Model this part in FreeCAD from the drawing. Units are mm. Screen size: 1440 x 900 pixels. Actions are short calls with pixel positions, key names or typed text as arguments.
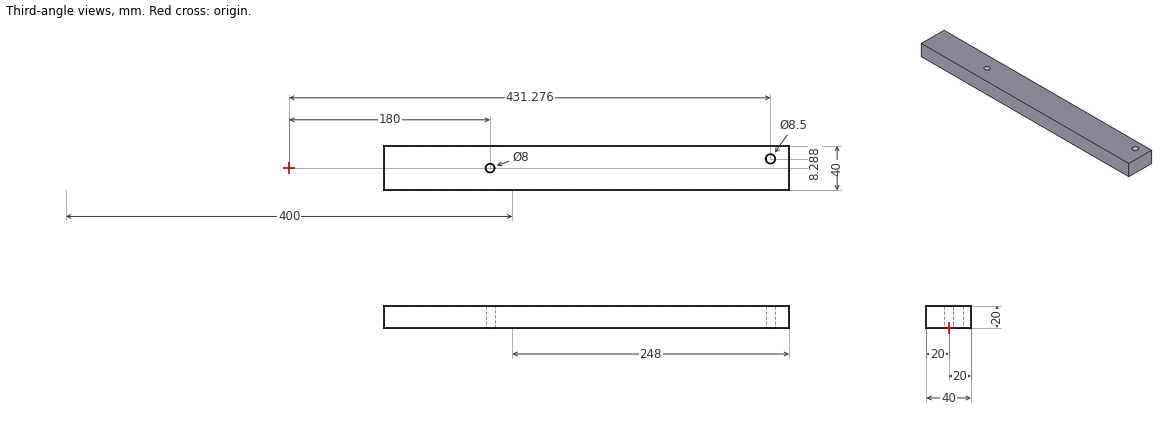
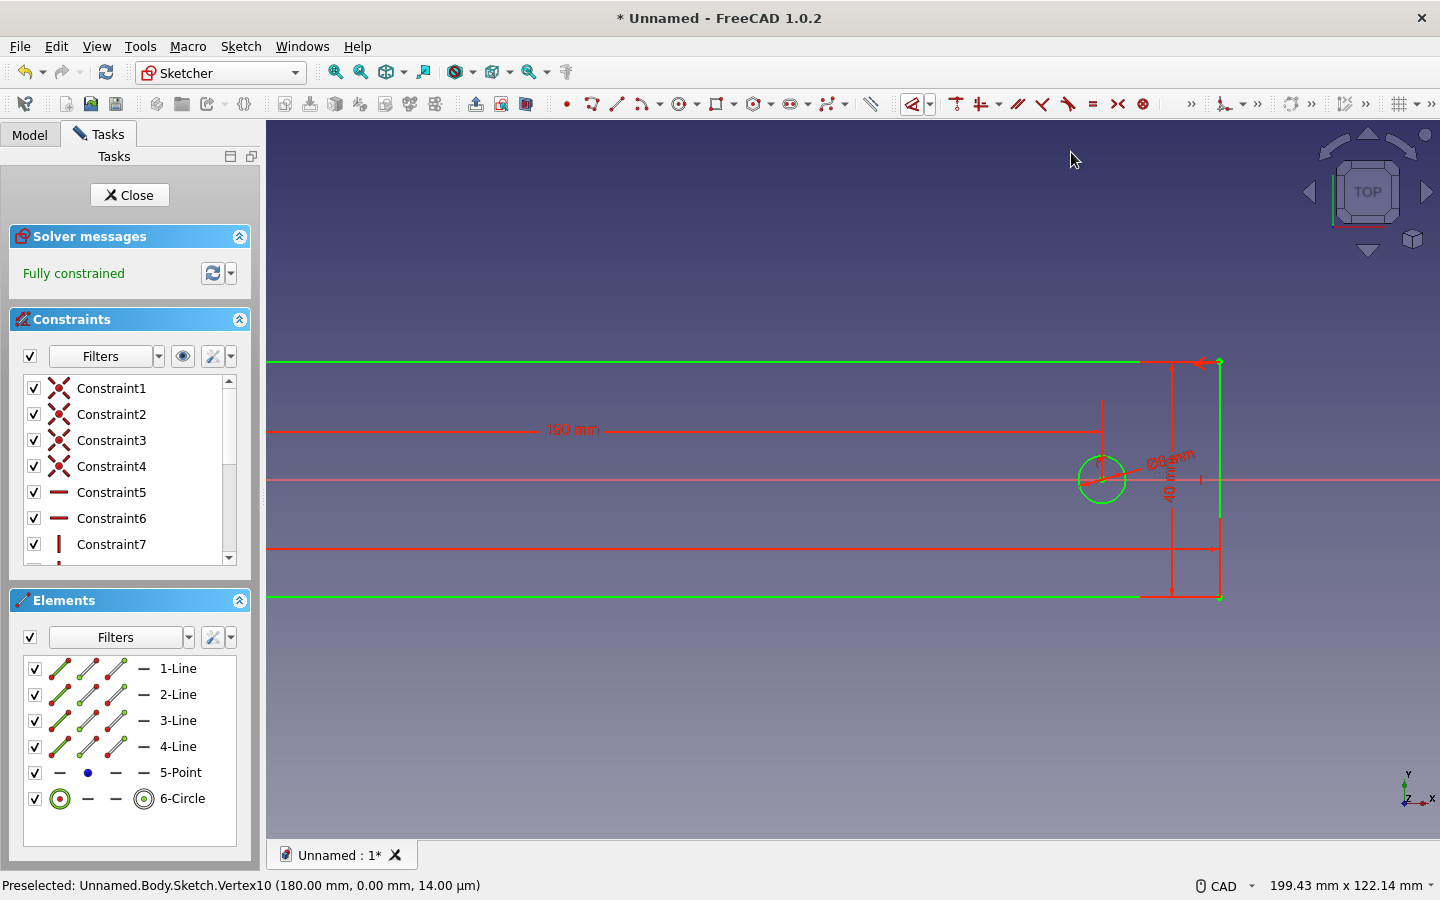
click(130, 195)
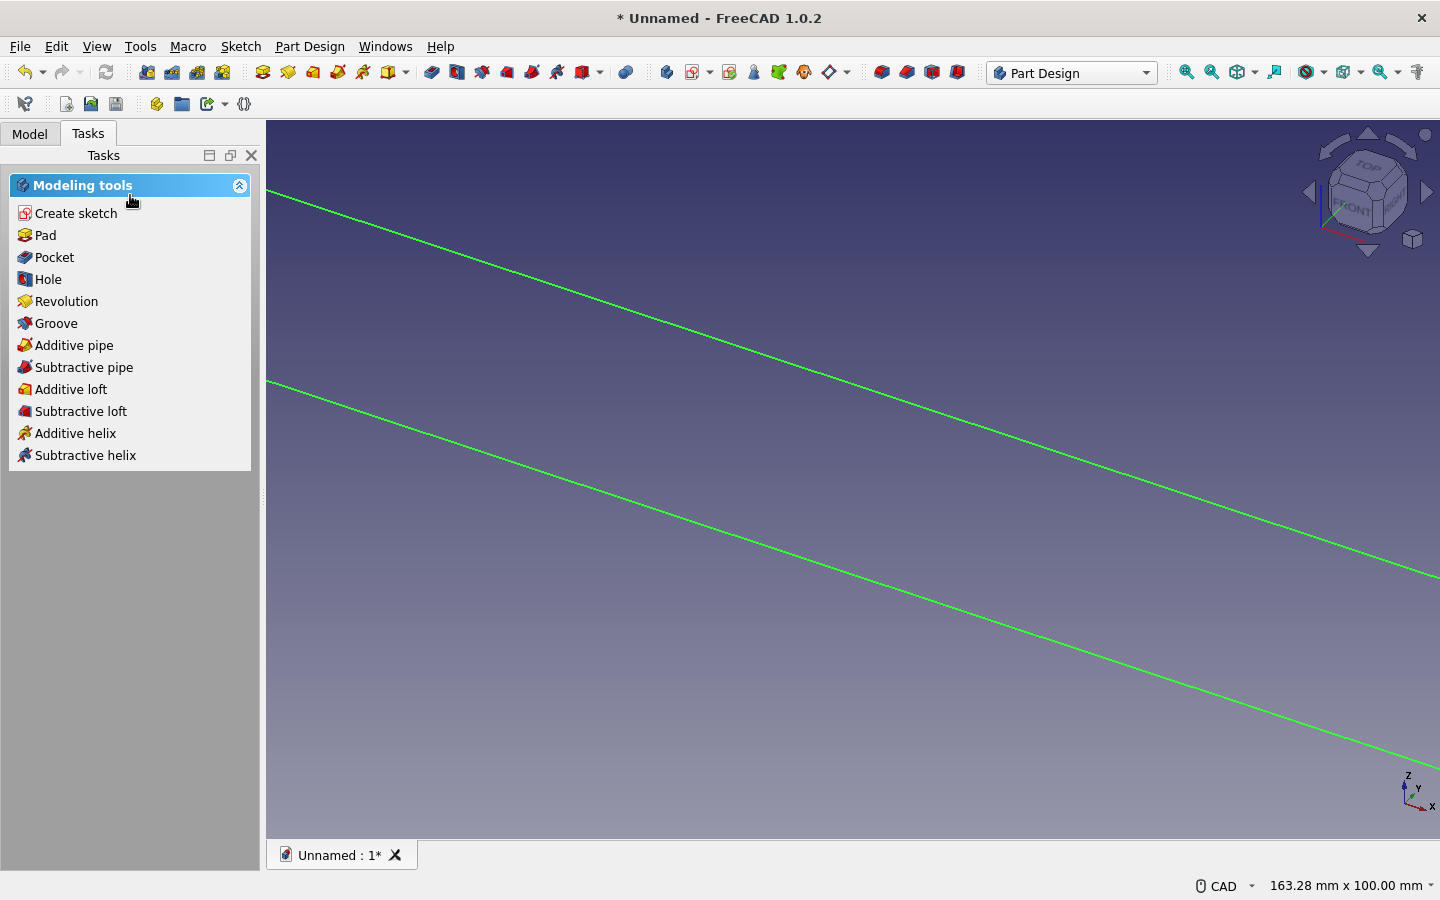
click(263, 72)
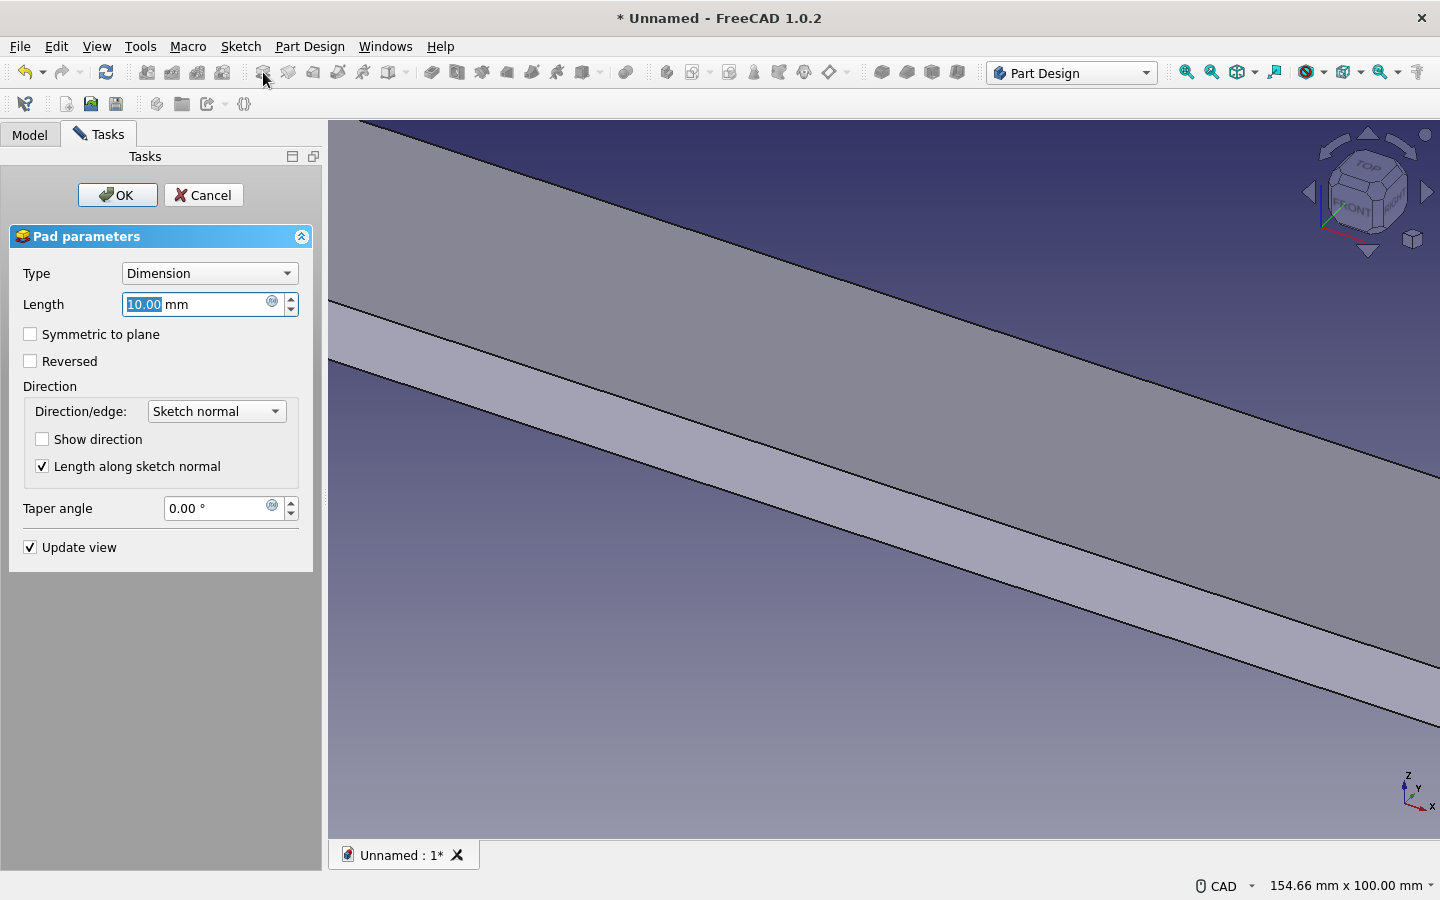
text(20)
key(Tab)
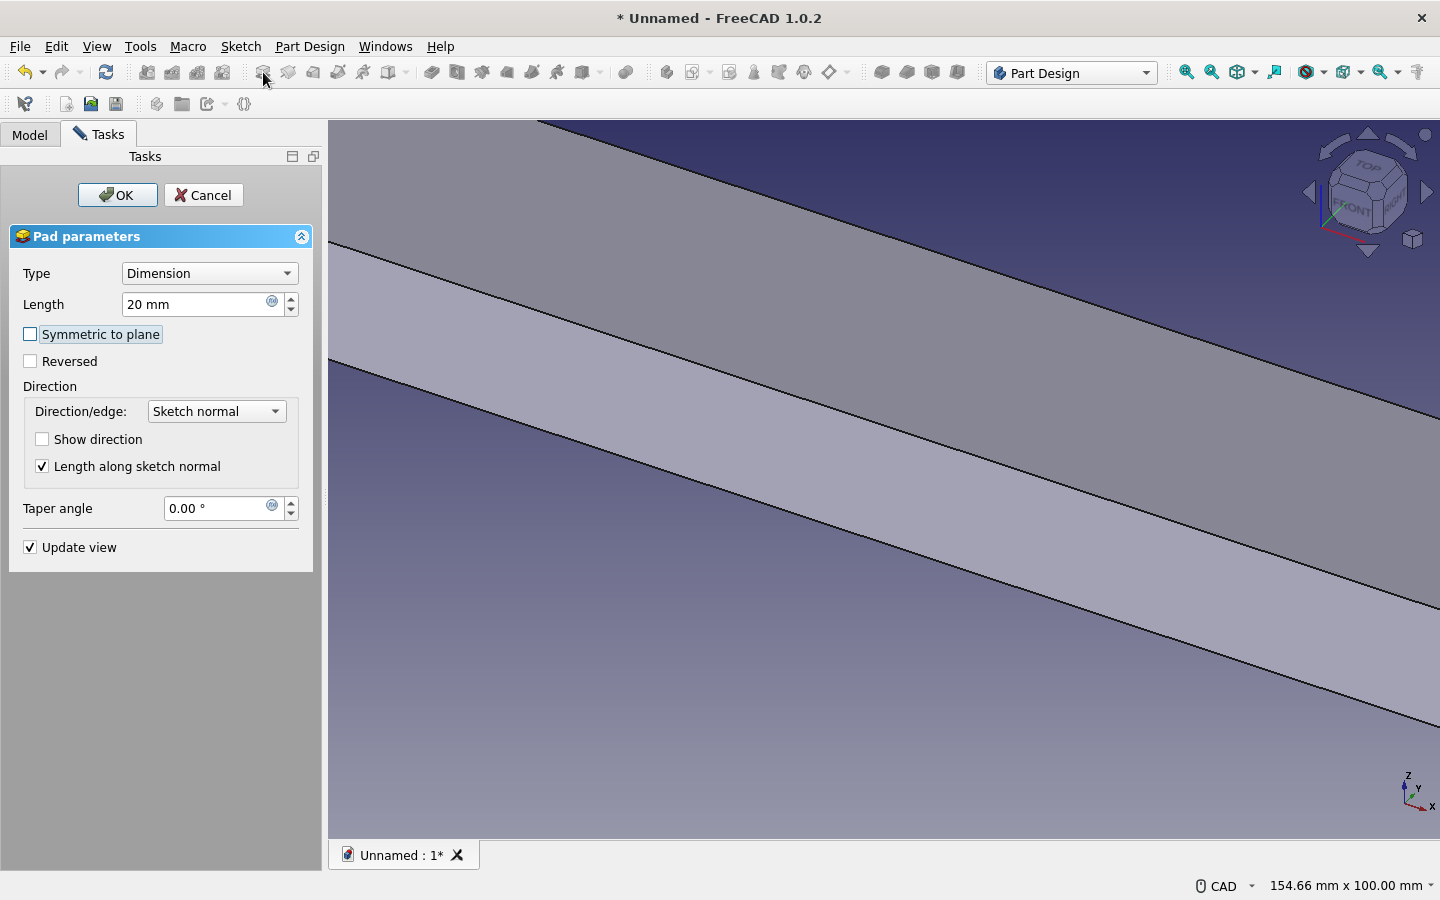
click(118, 195)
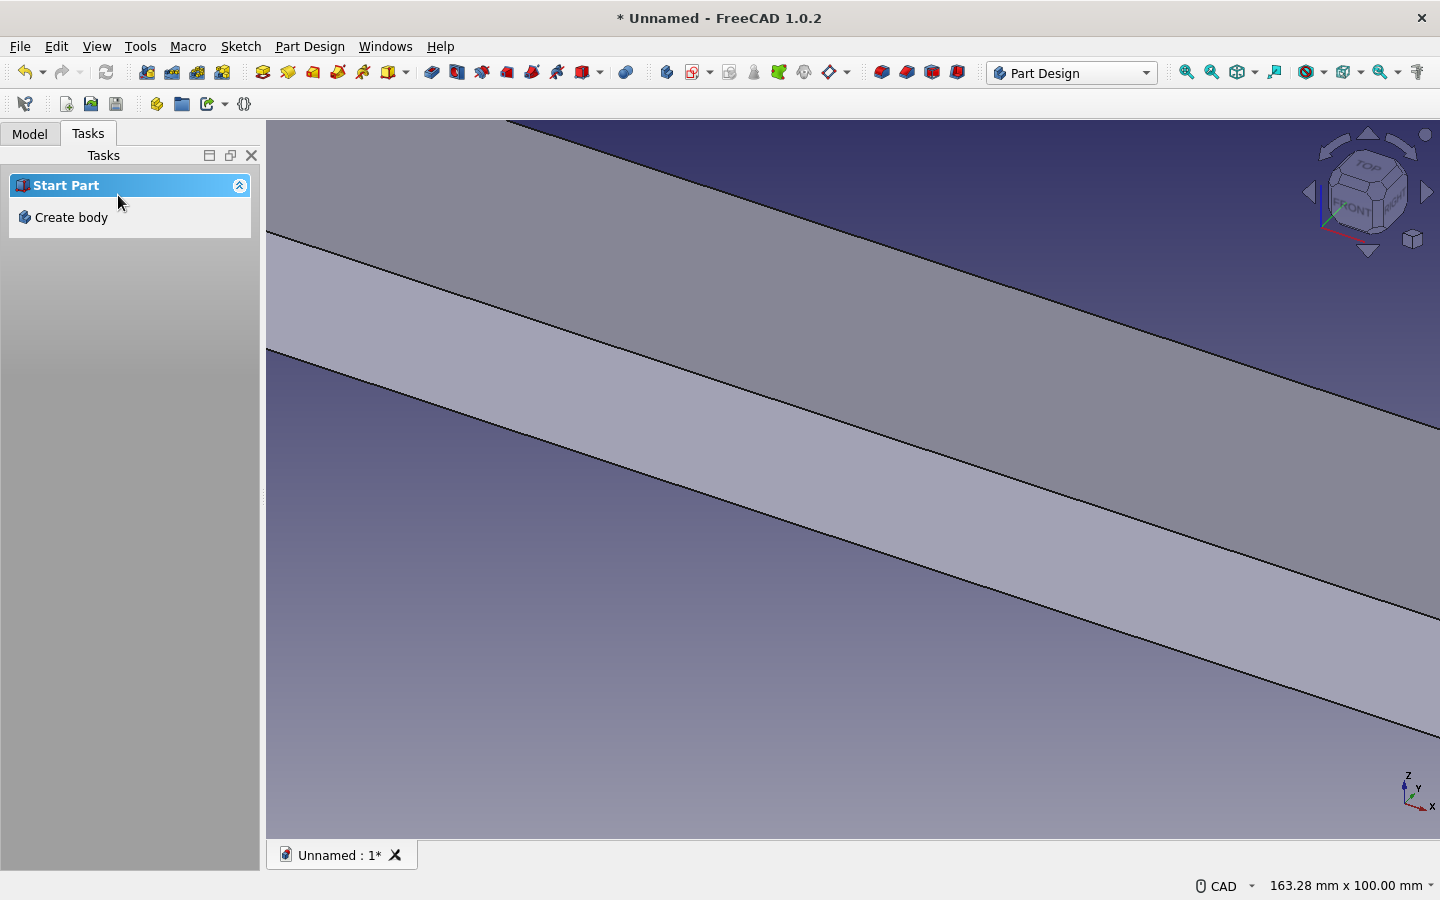
click(1187, 72)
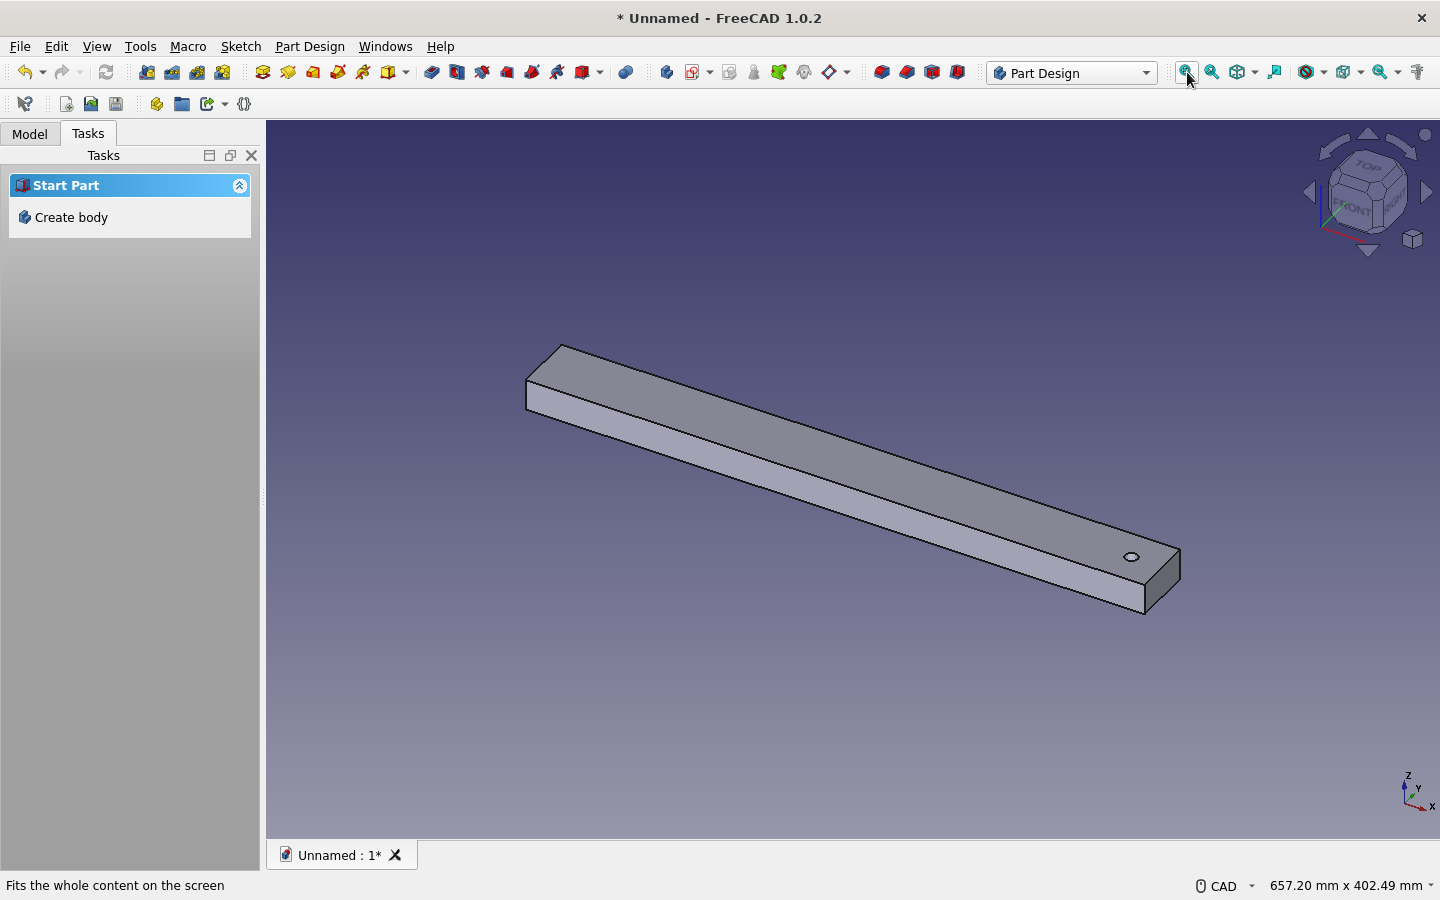
click(1168, 576)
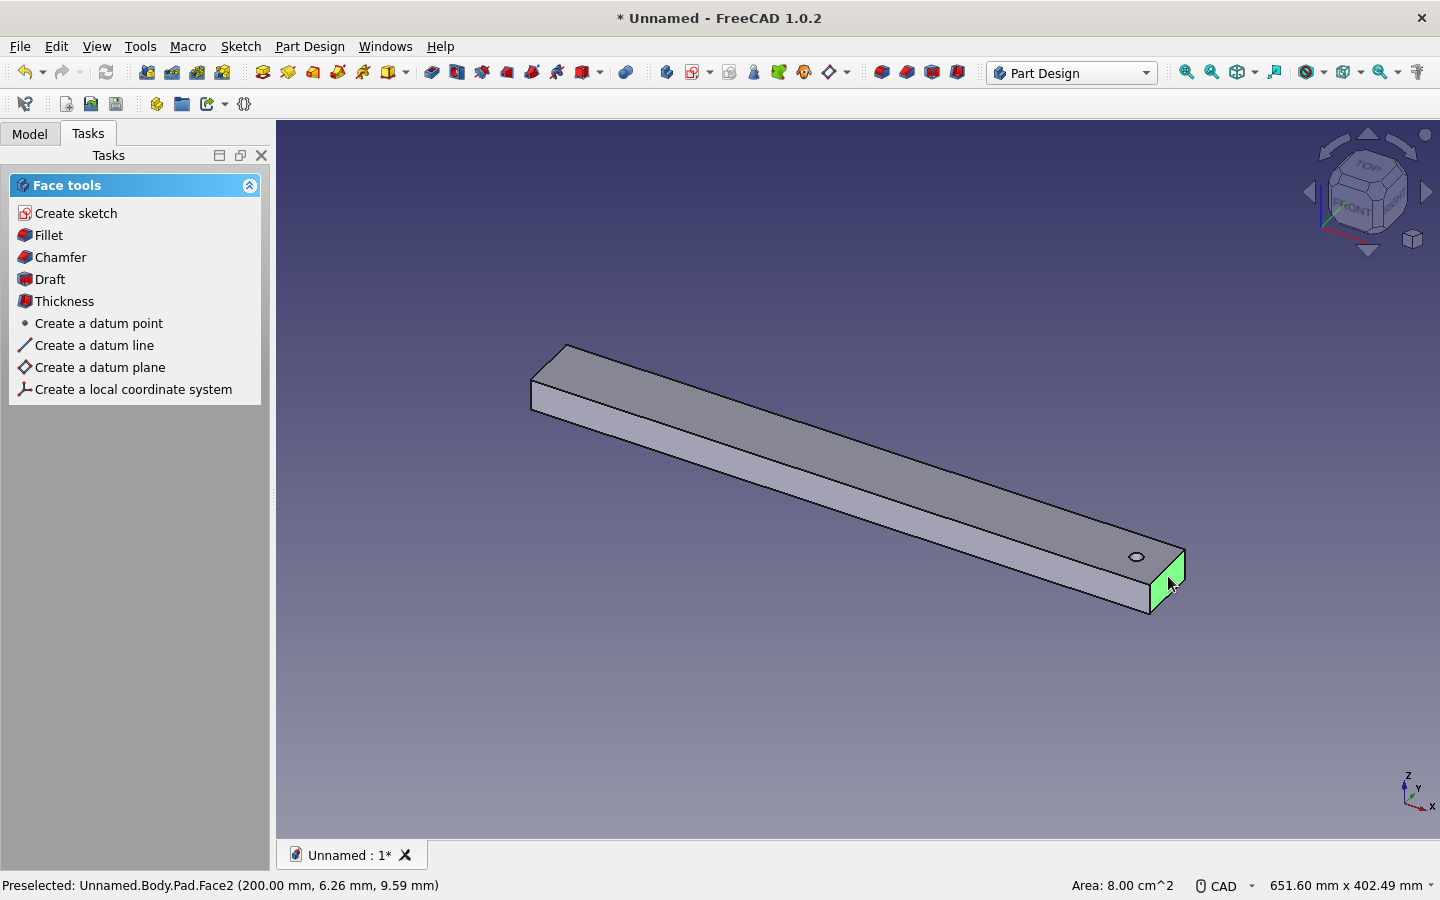
click(692, 72)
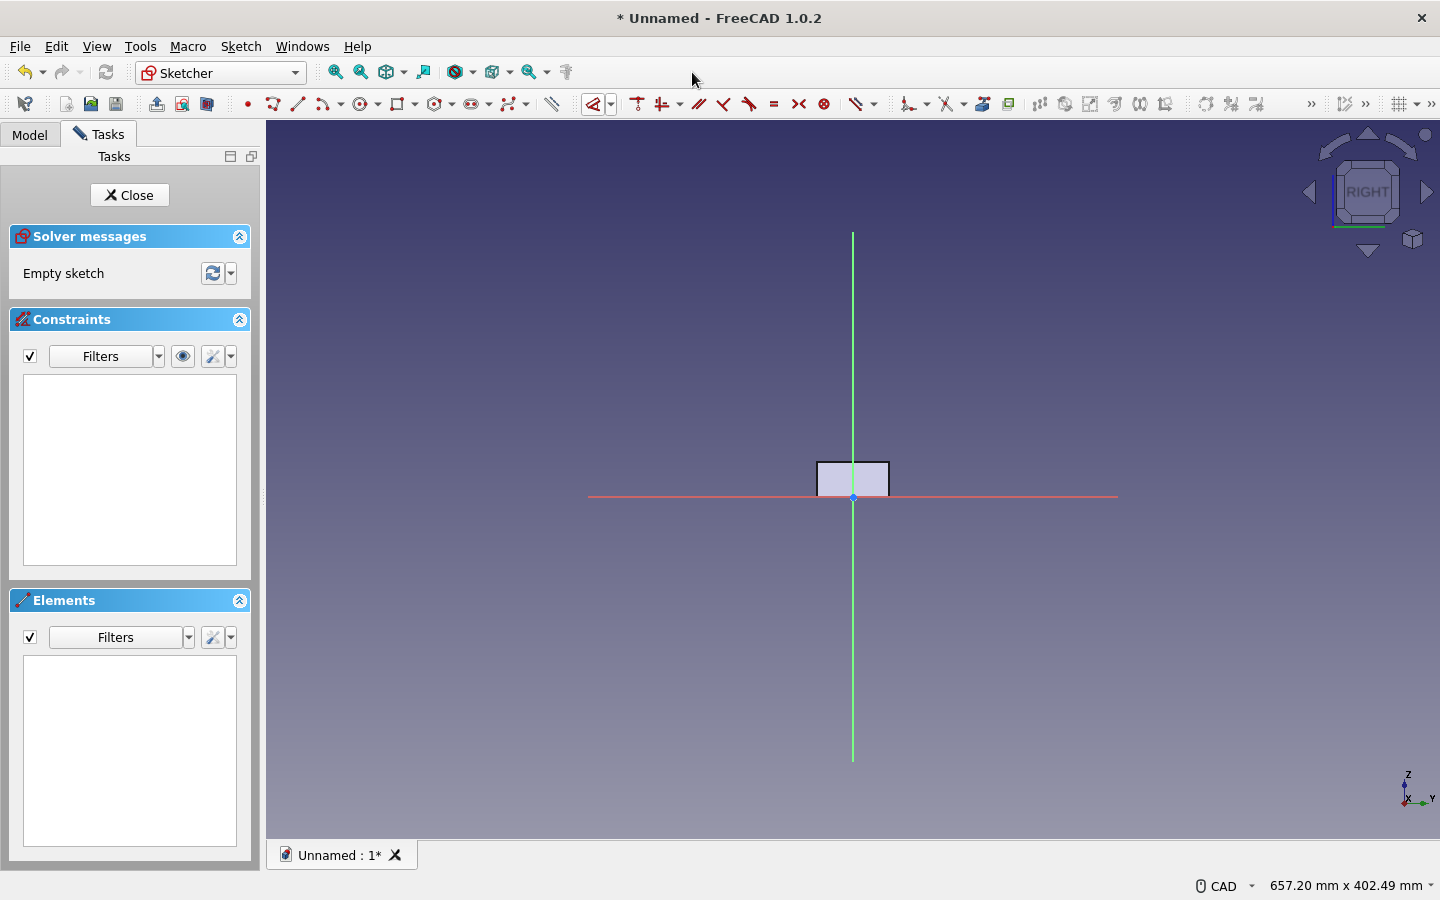
scroll(862, 479, up, 11)